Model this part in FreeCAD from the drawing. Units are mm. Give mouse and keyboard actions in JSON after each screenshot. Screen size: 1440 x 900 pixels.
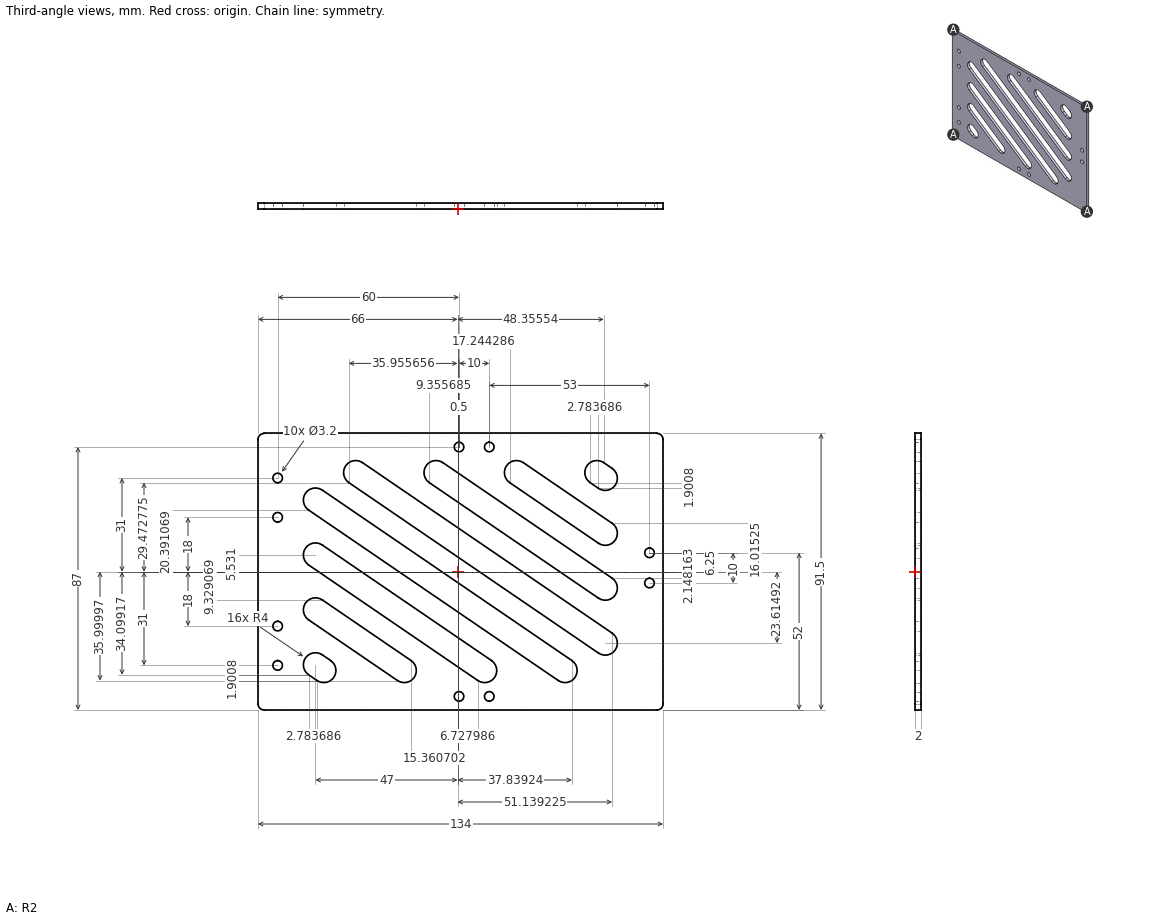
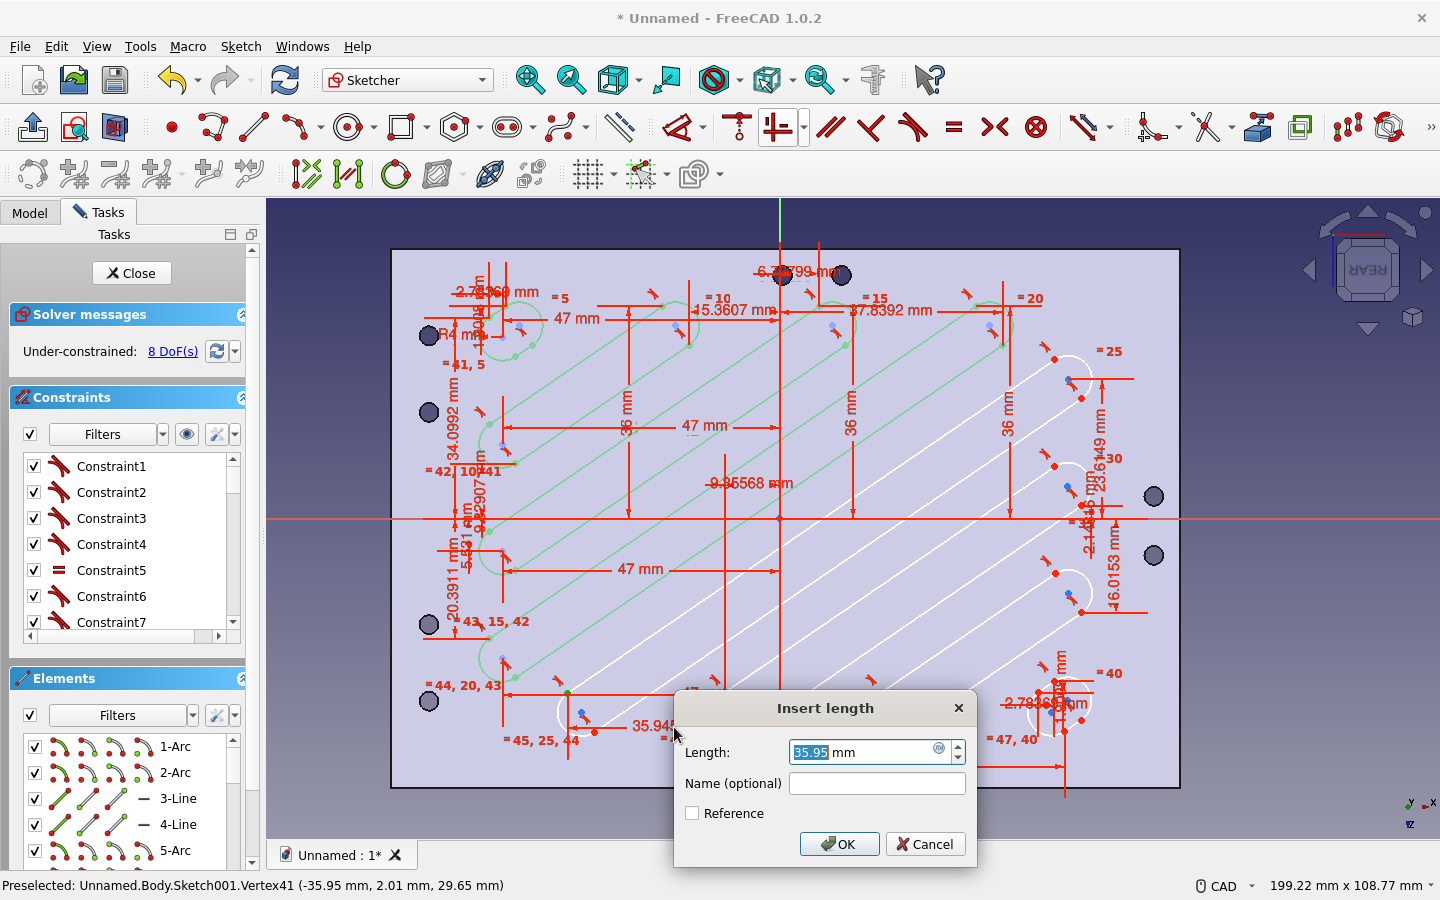
{"action": "type", "text": "35.955656"}
{"action": "key", "text": "Return"}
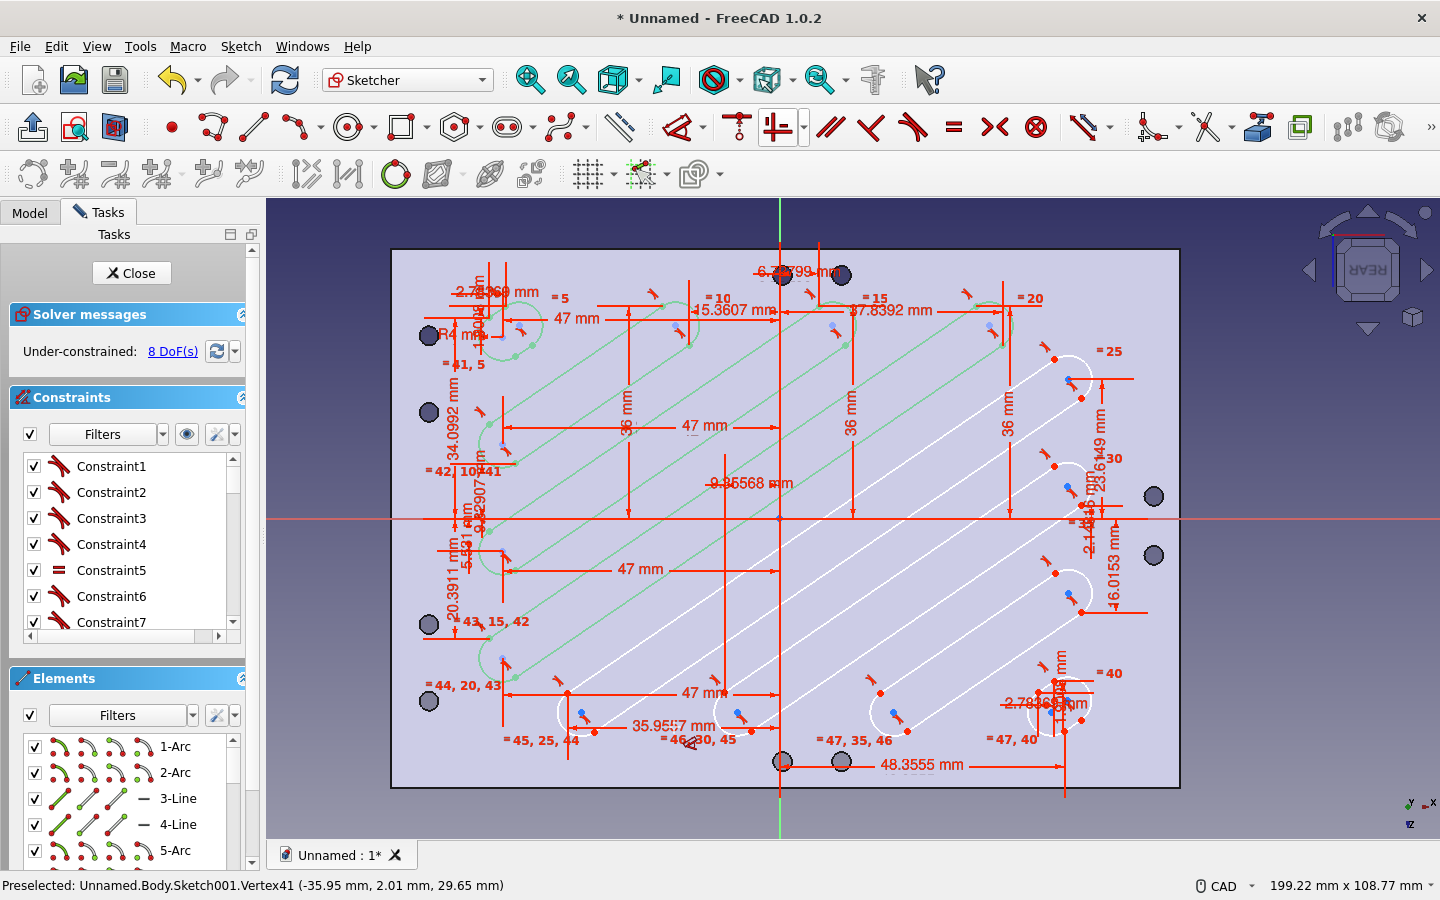
{"action": "left_click", "coordinate": [568, 693]}
{"action": "left_click", "coordinate": [534, 646]}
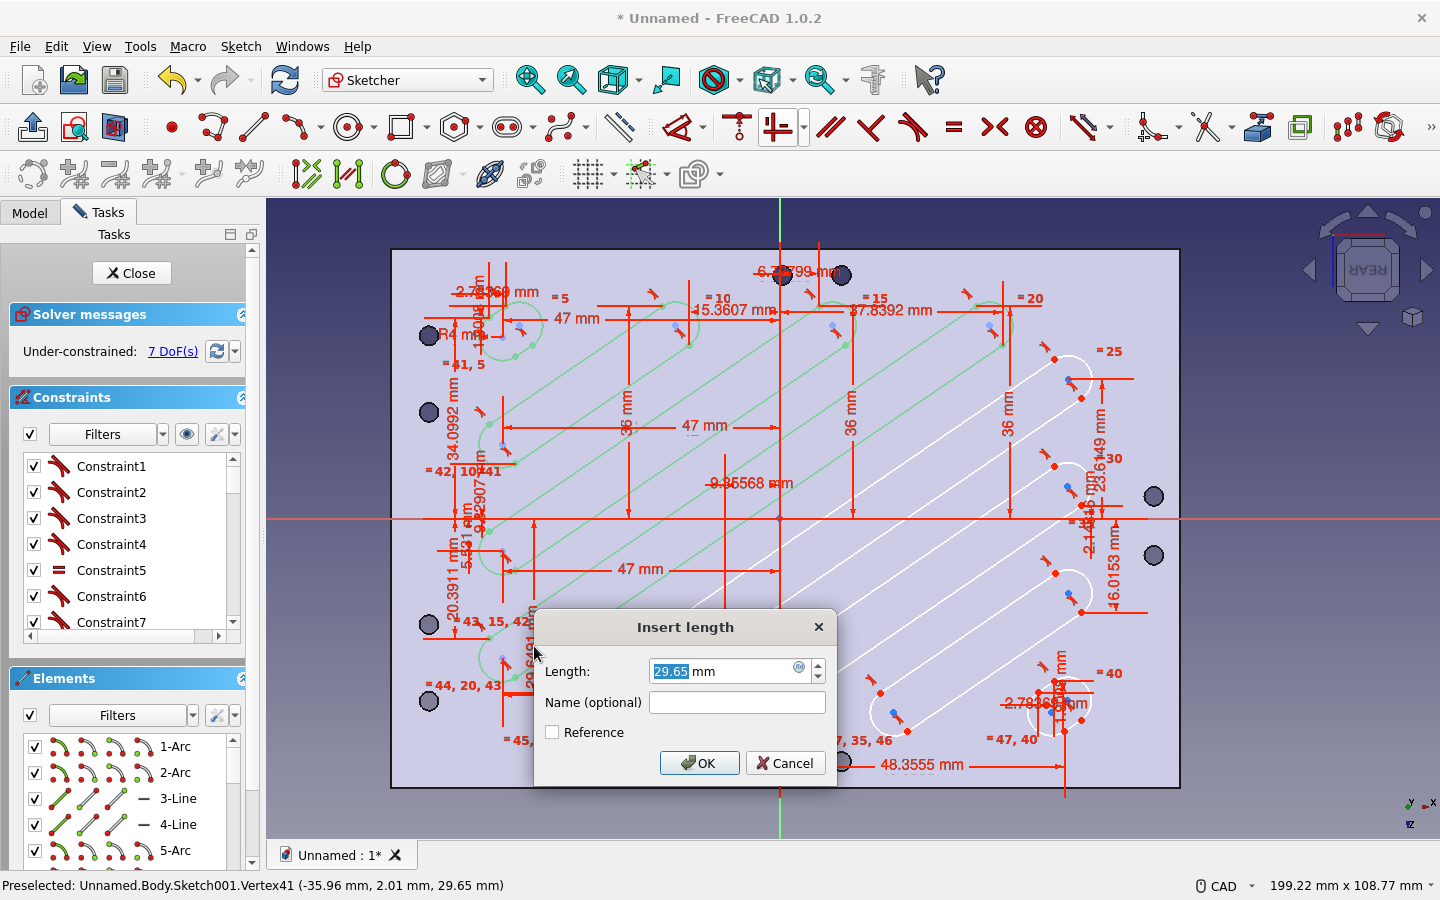
{"action": "type", "text": "29.472775"}
{"action": "key", "text": "Return"}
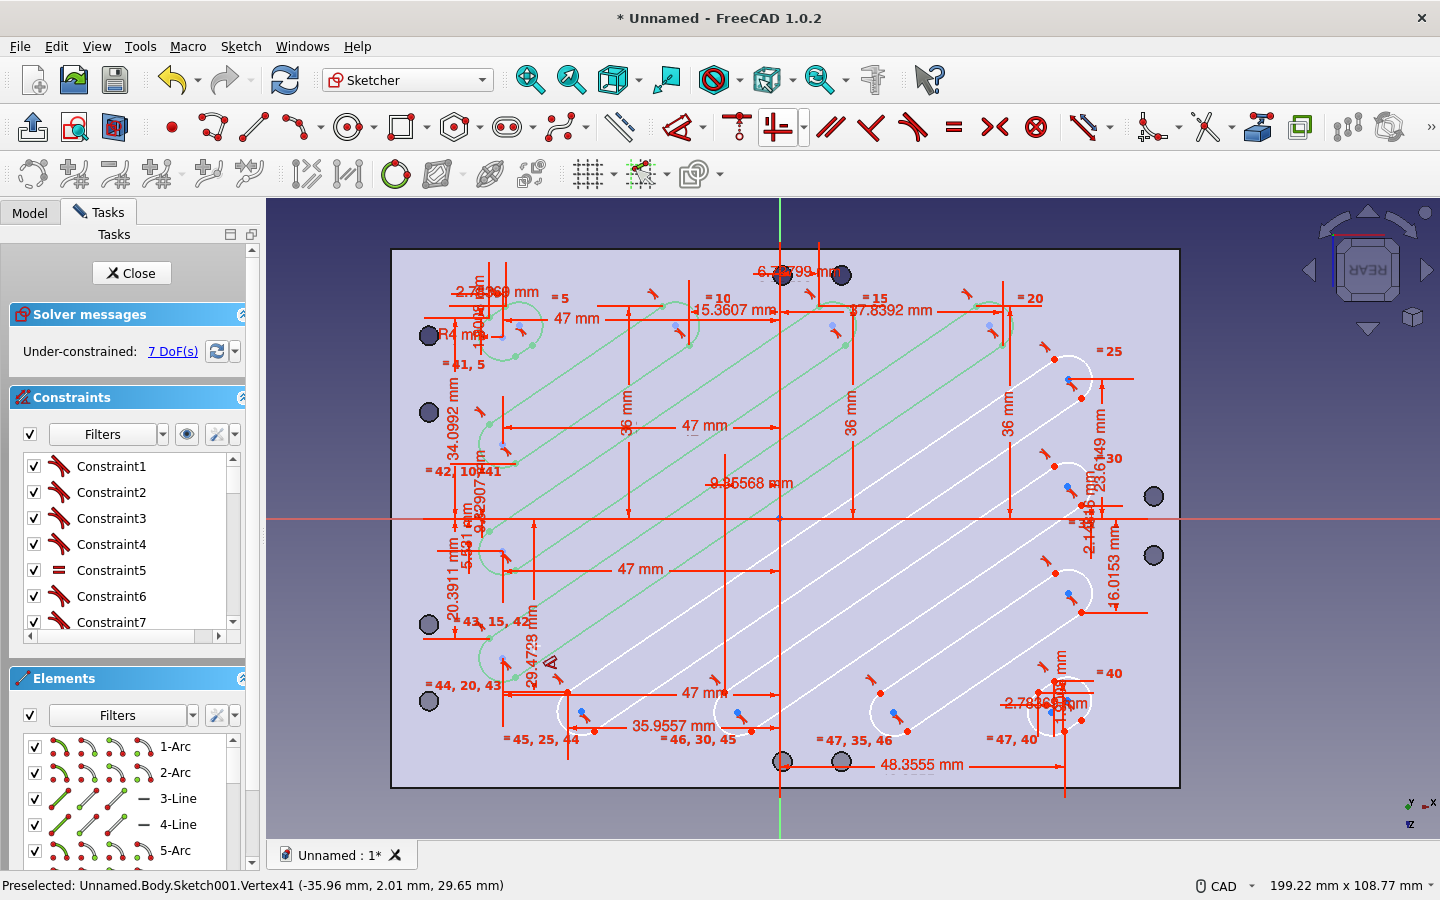
{"action": "left_click", "coordinate": [1082, 399]}
{"action": "left_click", "coordinate": [931, 365]}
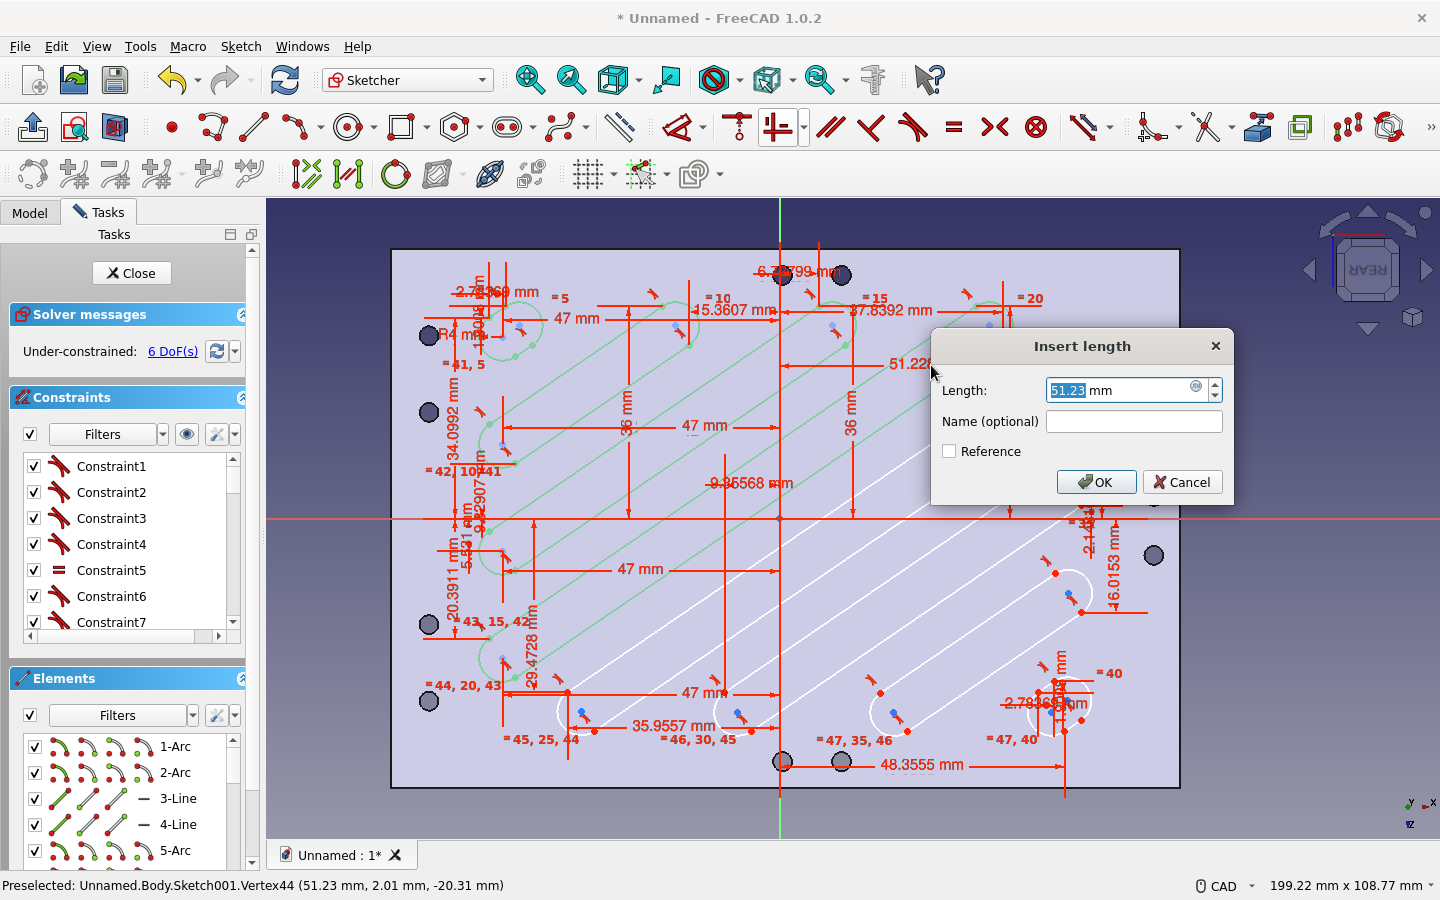
{"action": "type", "text": "51.139225"}
{"action": "key", "text": "Return"}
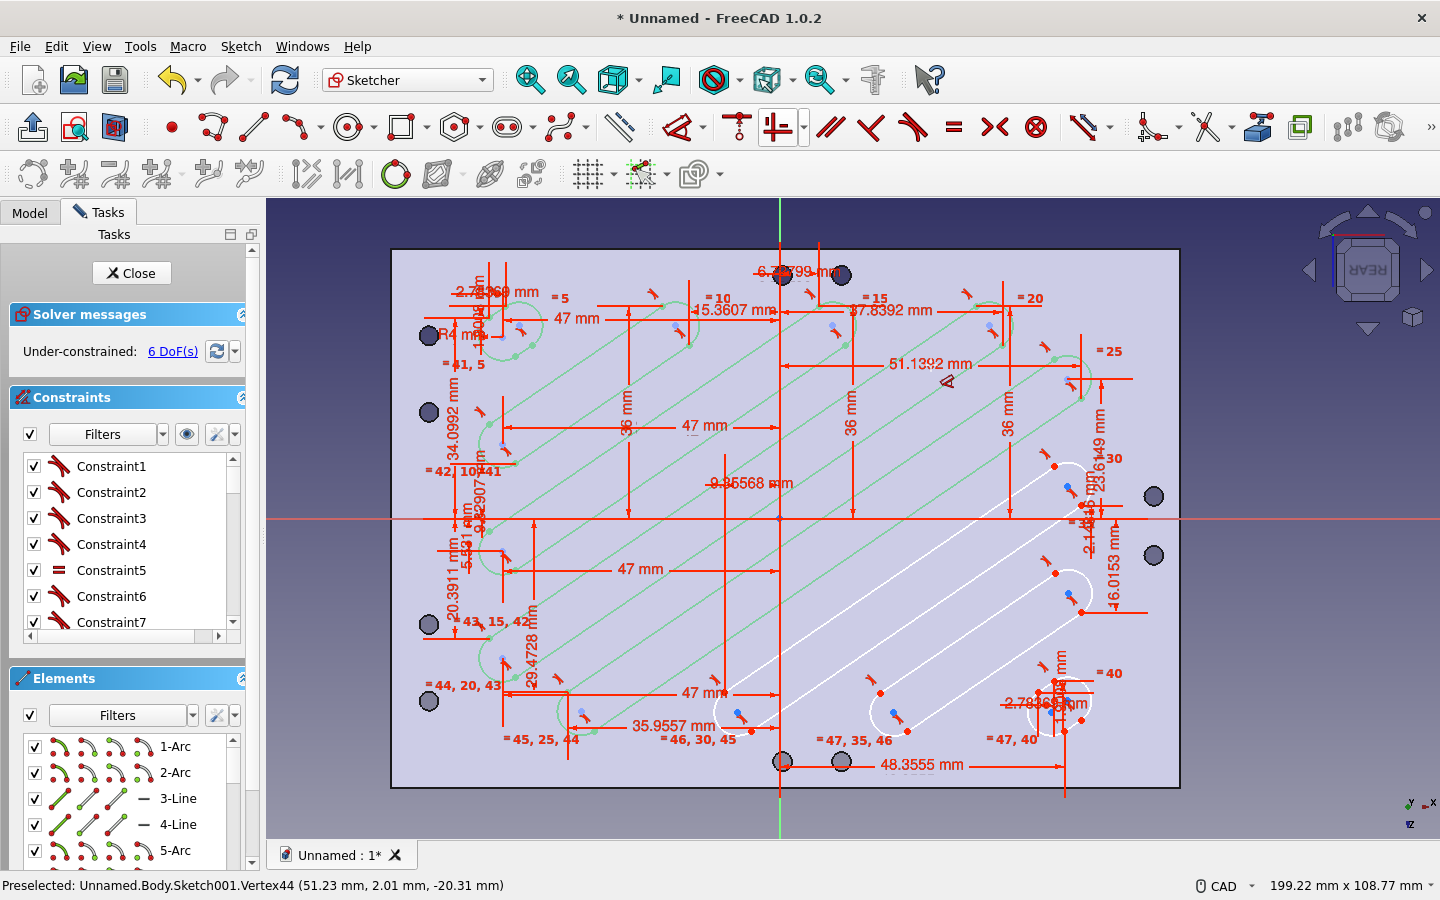
{"action": "left_click", "coordinate": [725, 693]}
{"action": "left_click", "coordinate": [691, 646]}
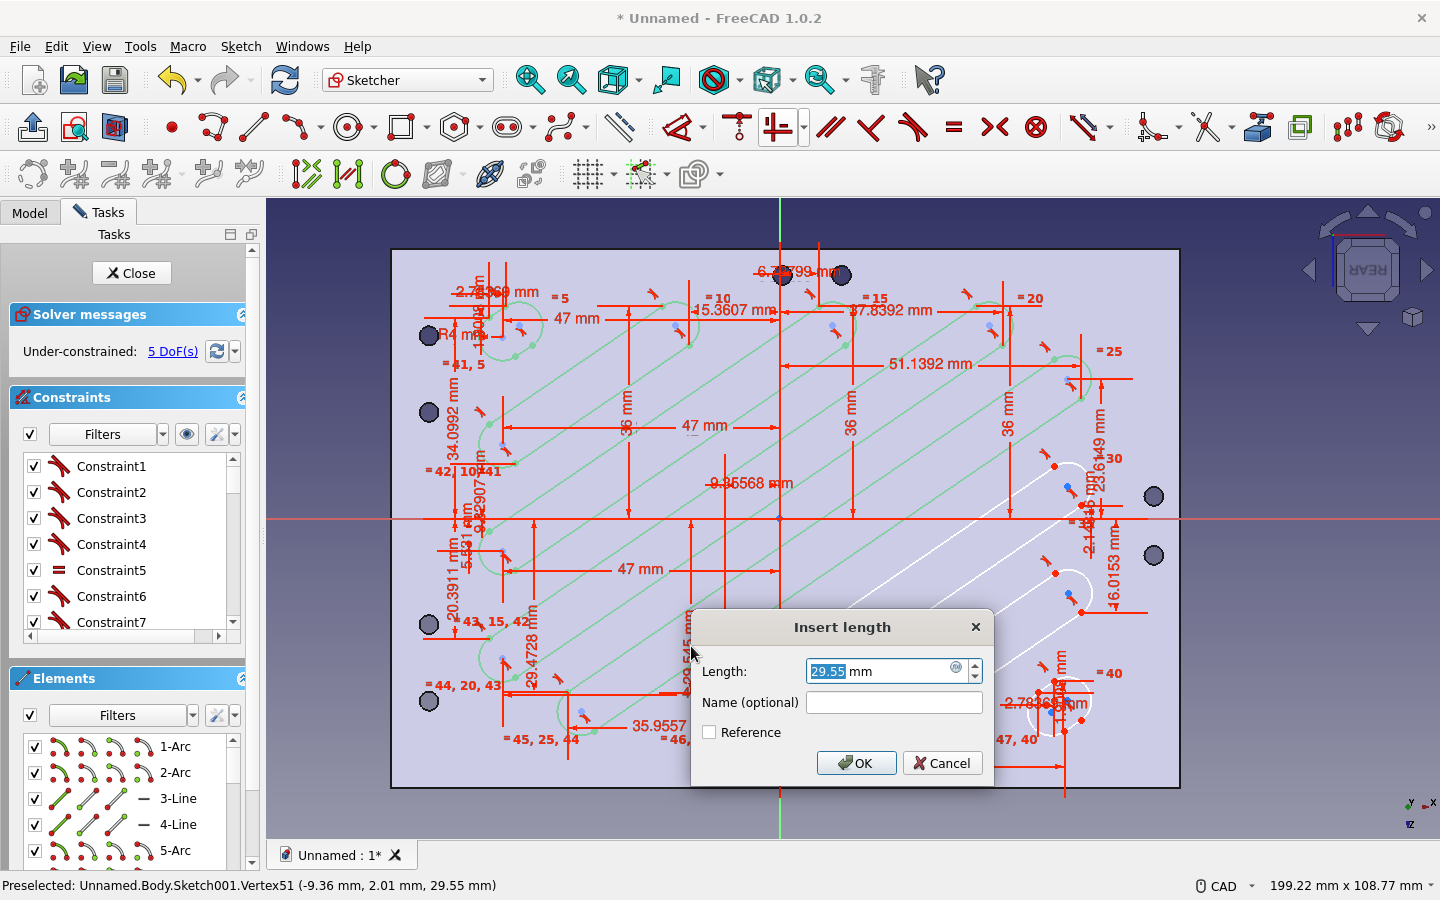
{"action": "type", "text": "29.472775"}
{"action": "key", "text": "Return"}